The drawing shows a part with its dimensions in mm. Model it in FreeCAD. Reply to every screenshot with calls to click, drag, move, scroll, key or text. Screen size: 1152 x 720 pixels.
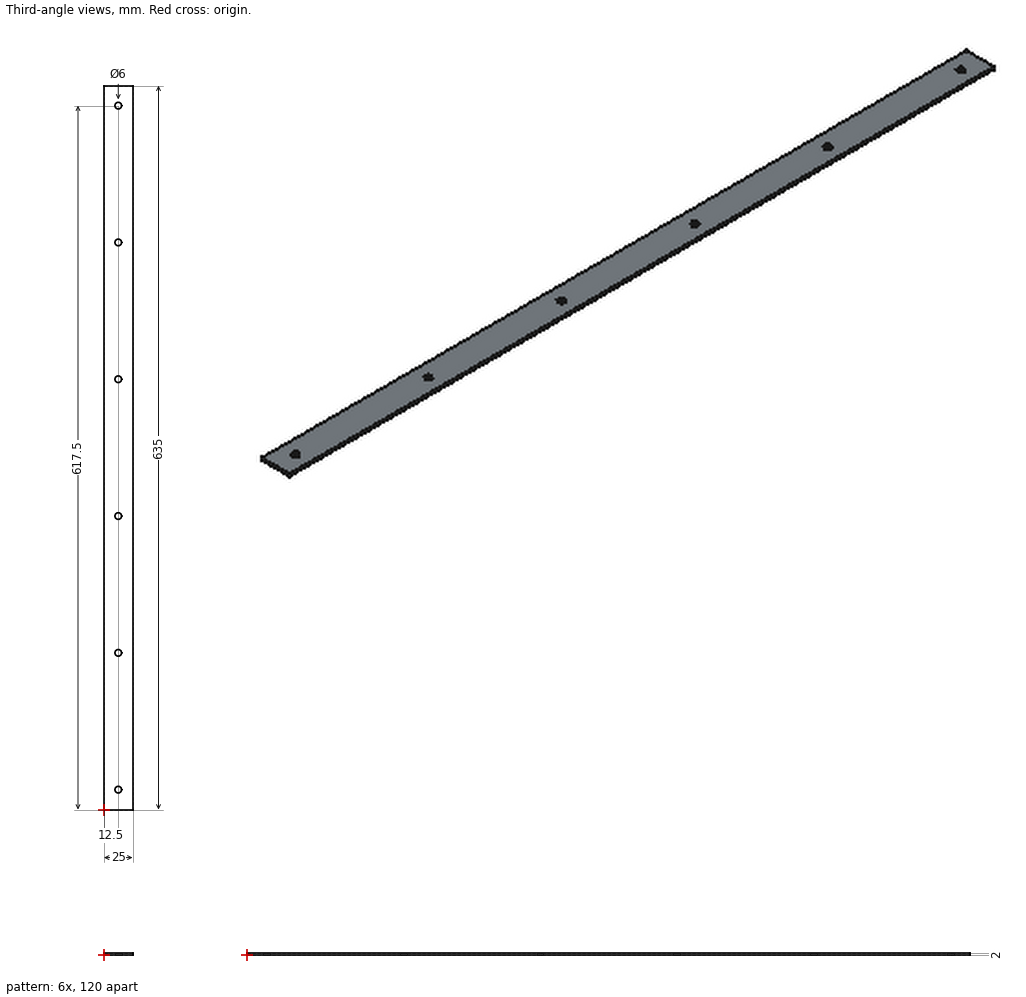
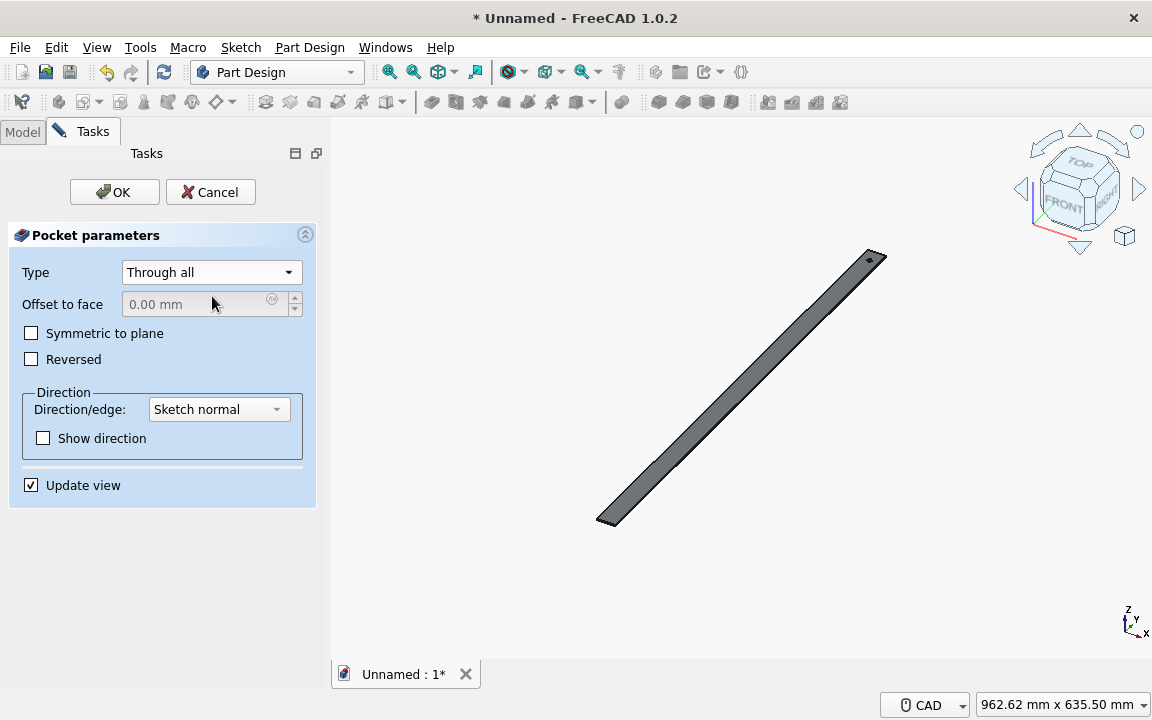
click(115, 192)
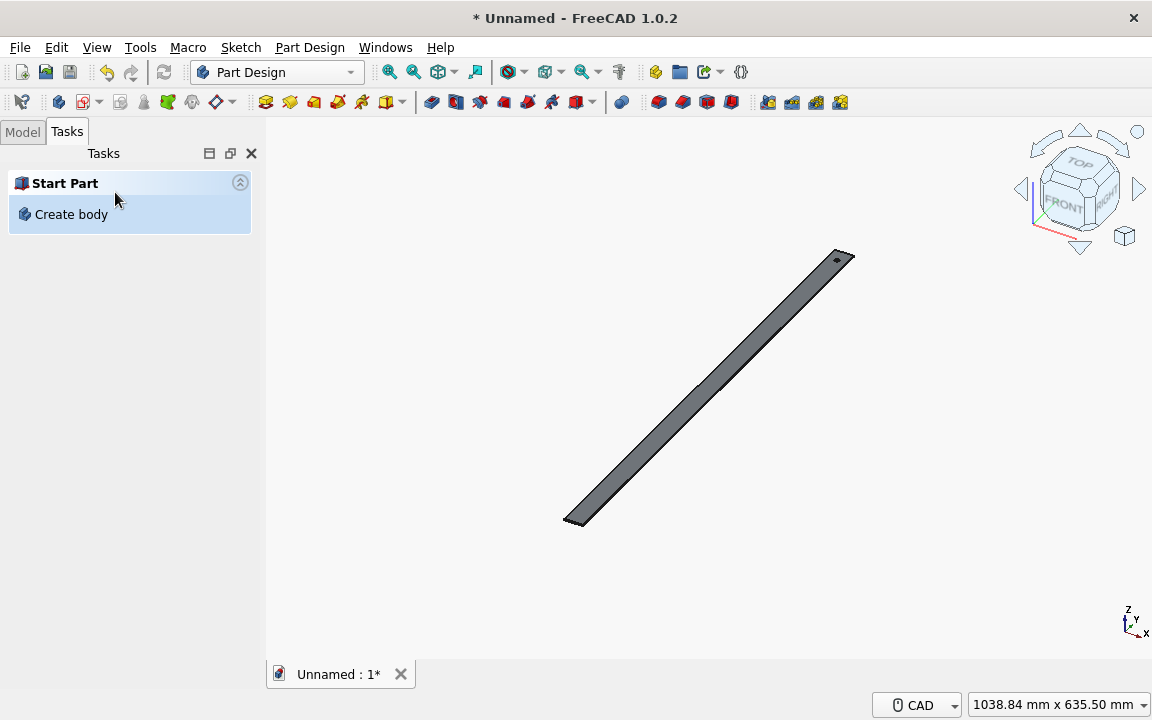
click(23, 131)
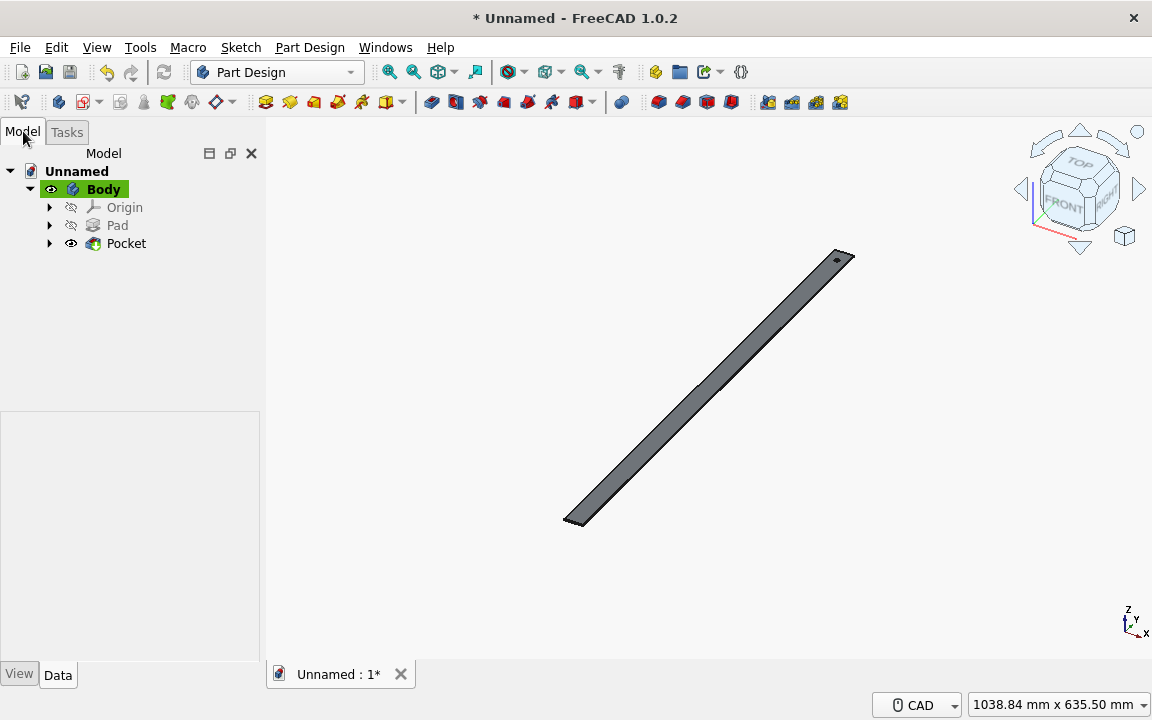
click(116, 243)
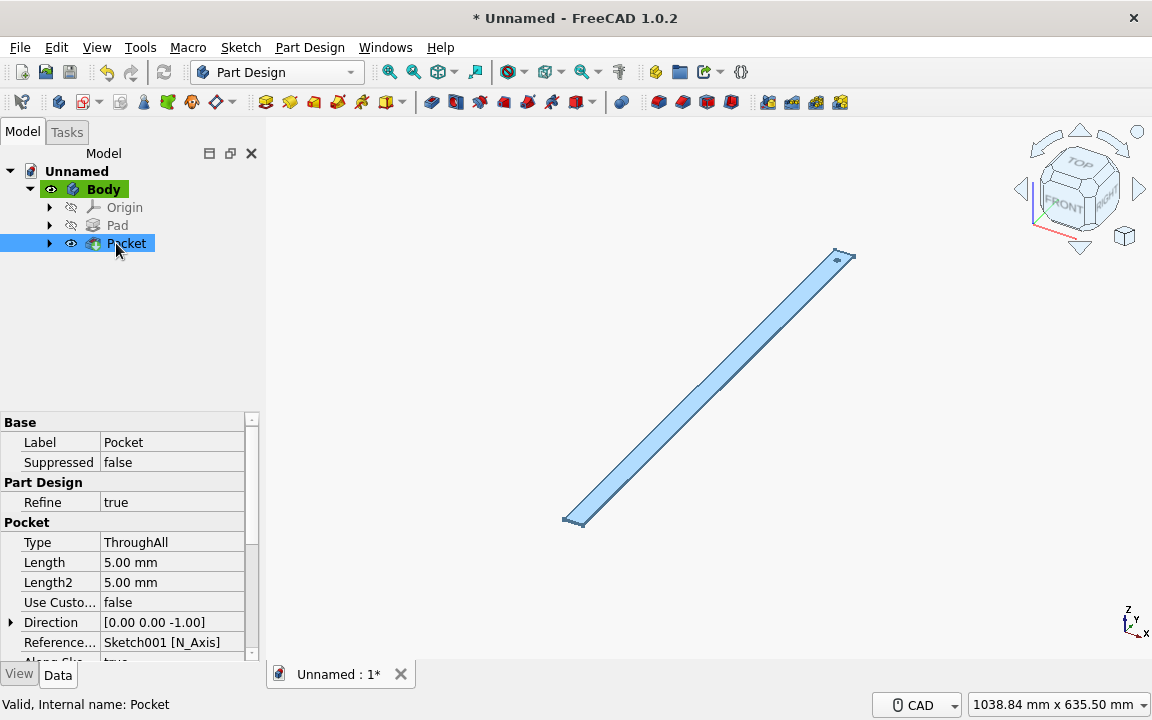
click(792, 102)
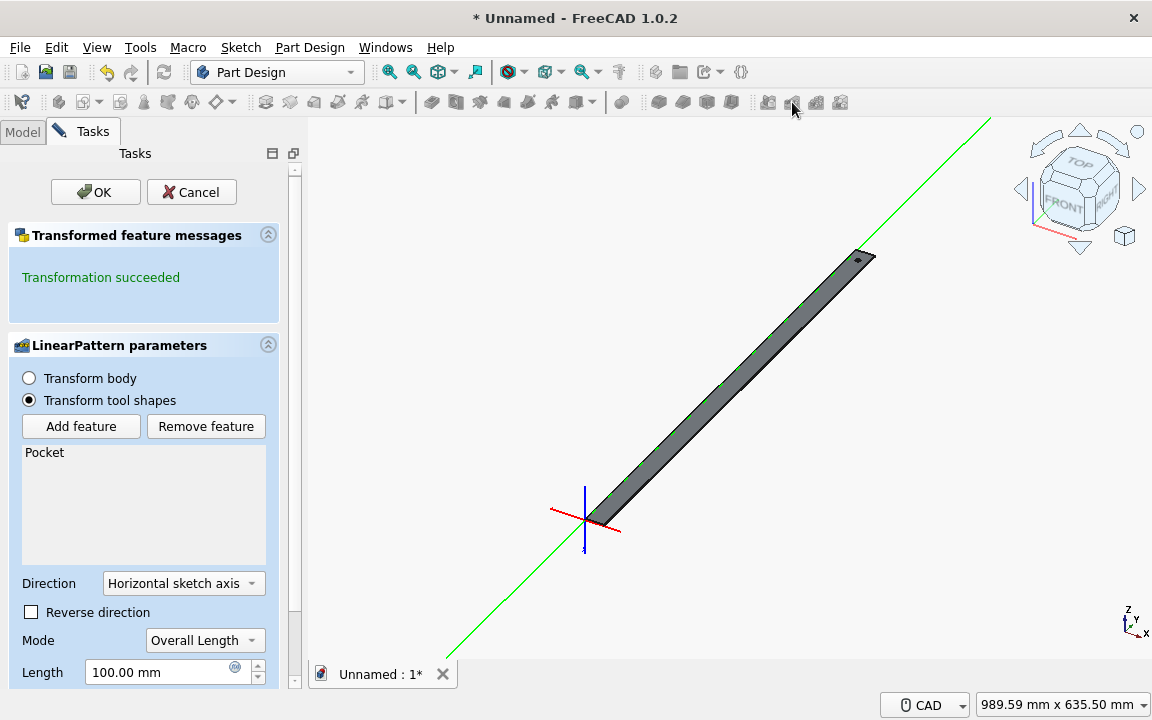
click(184, 584)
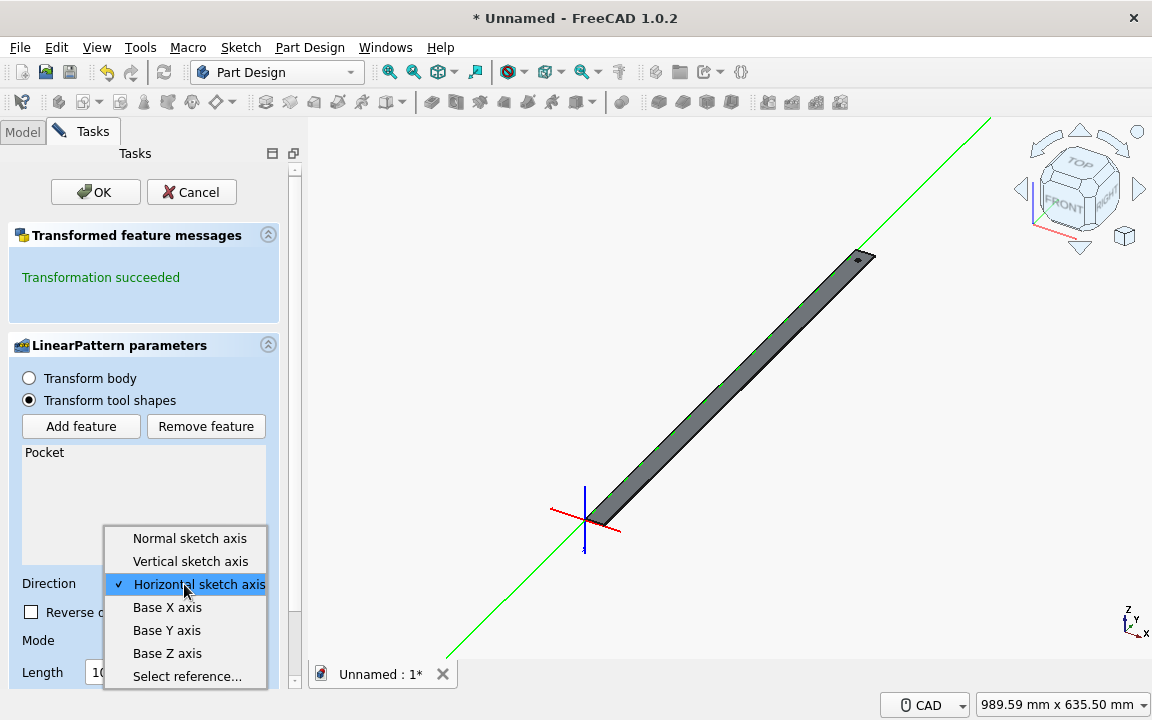
click(184, 630)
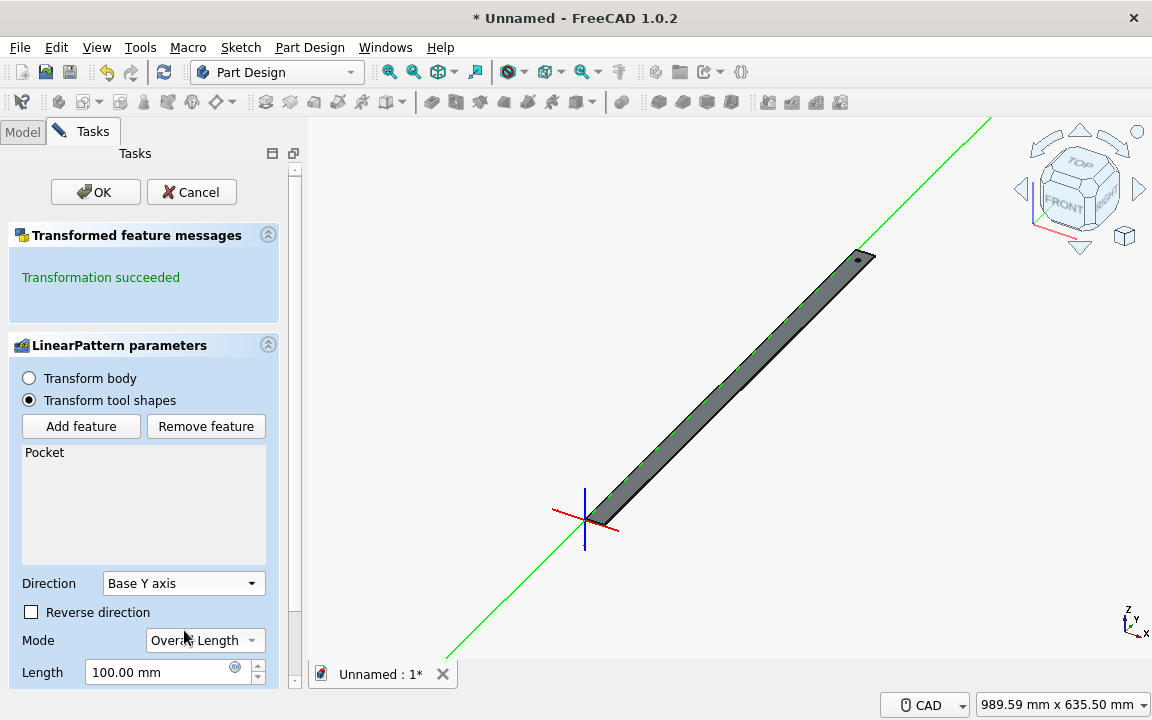
click(206, 640)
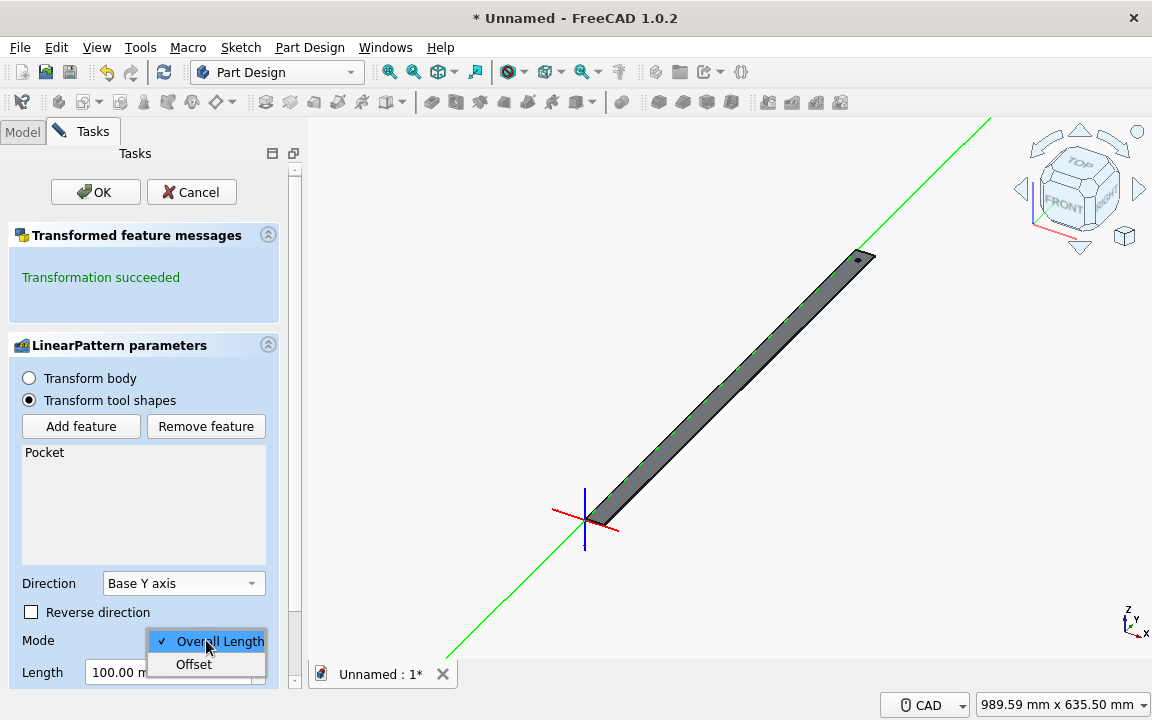
click(206, 664)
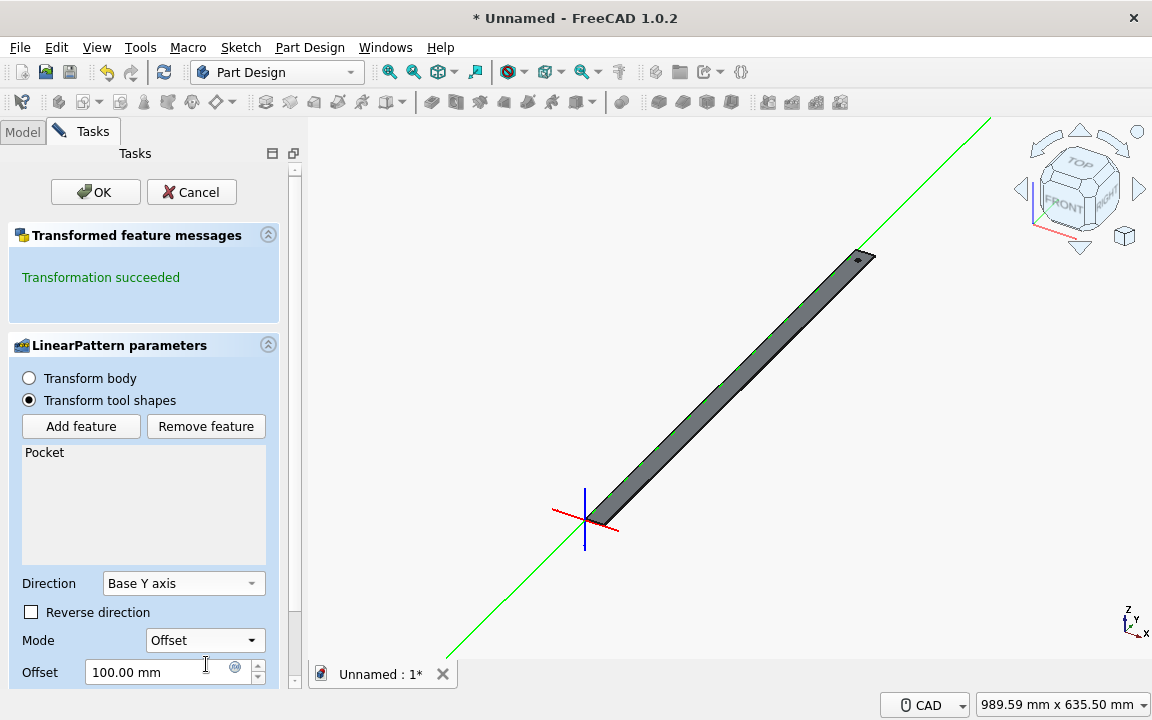
triple_click(168, 672)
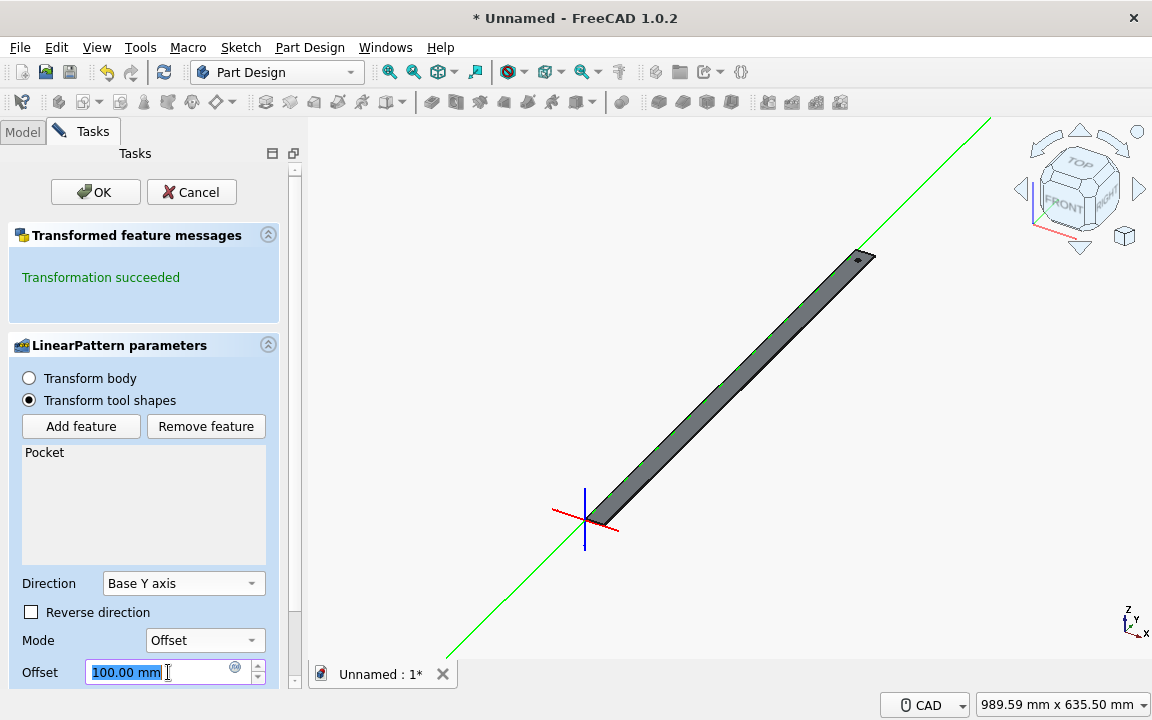
text(120)
key(Tab)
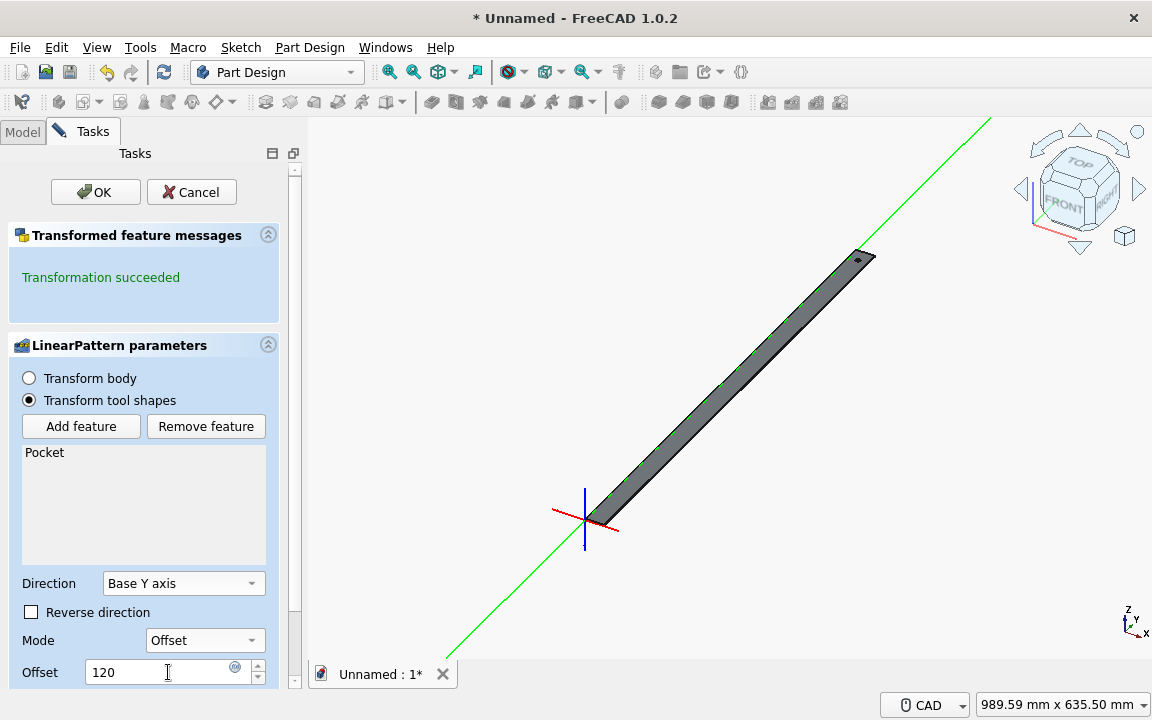
scroll(295, 426, down, 2)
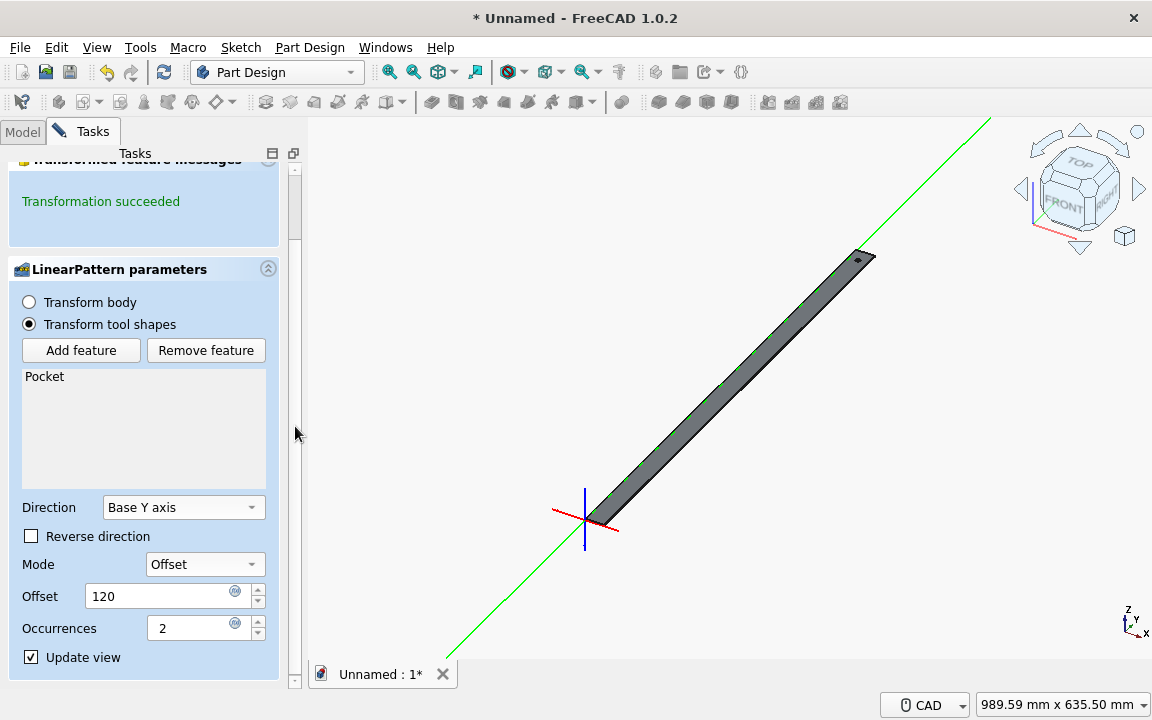
triple_click(198, 628)